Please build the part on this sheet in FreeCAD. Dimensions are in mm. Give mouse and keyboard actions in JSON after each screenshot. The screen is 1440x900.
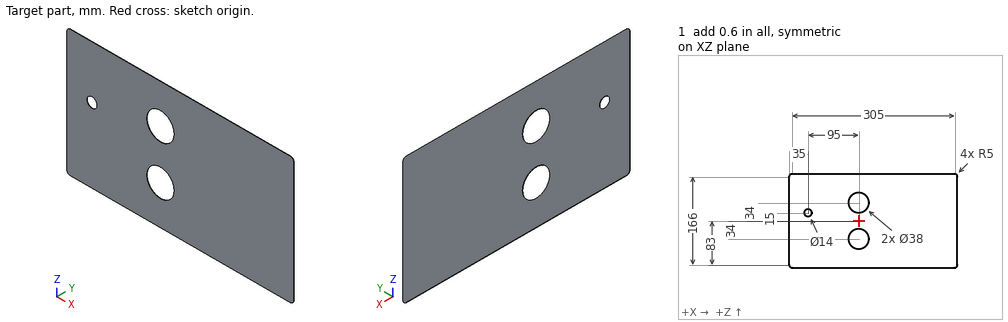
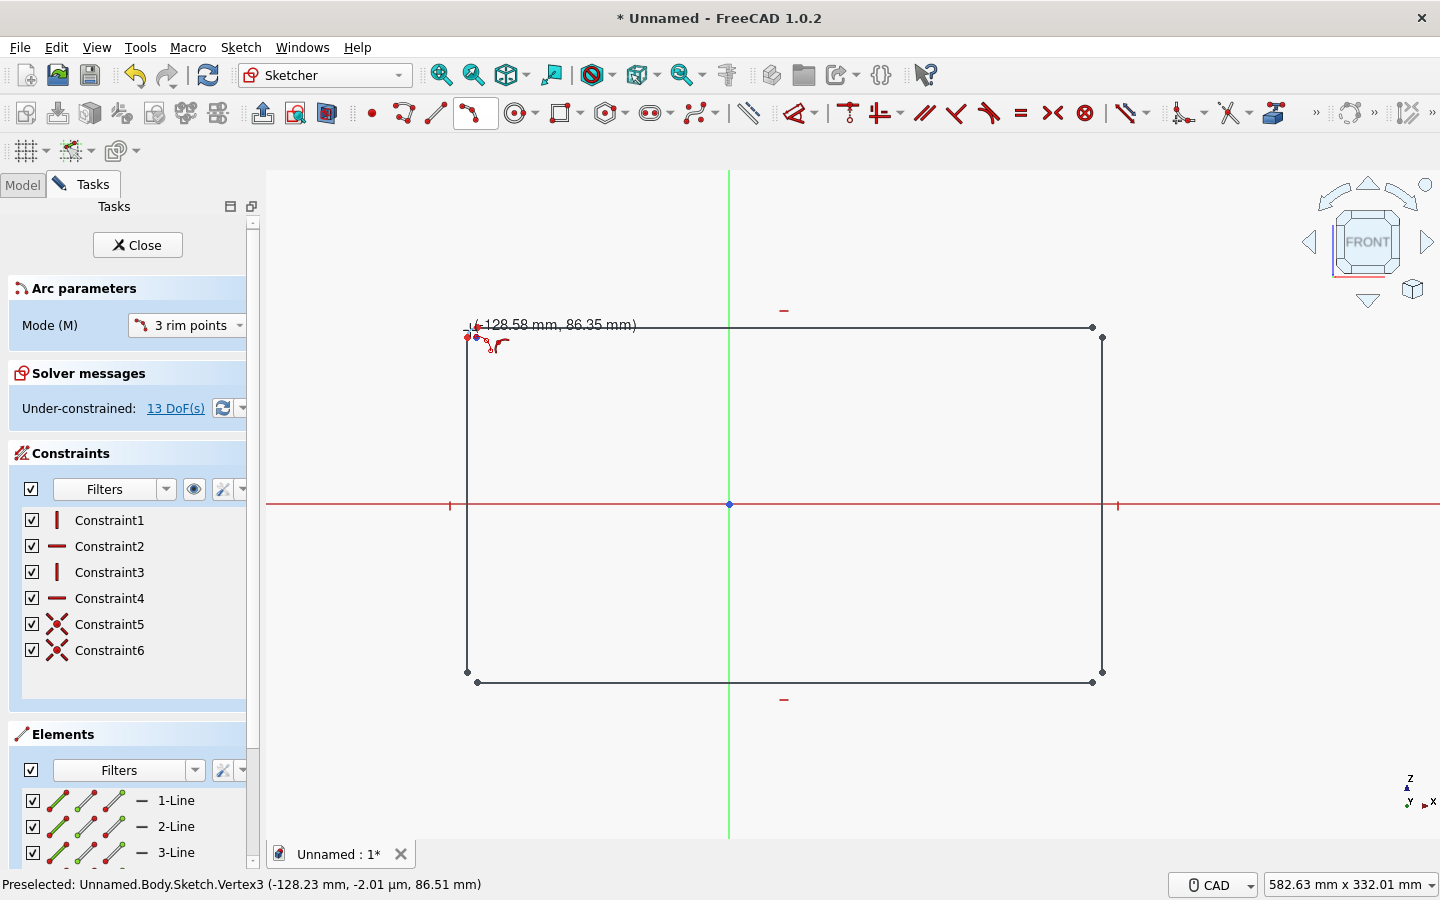
{"action": "left_click", "coordinate": [1092, 328]}
{"action": "left_click", "coordinate": [1102, 338]}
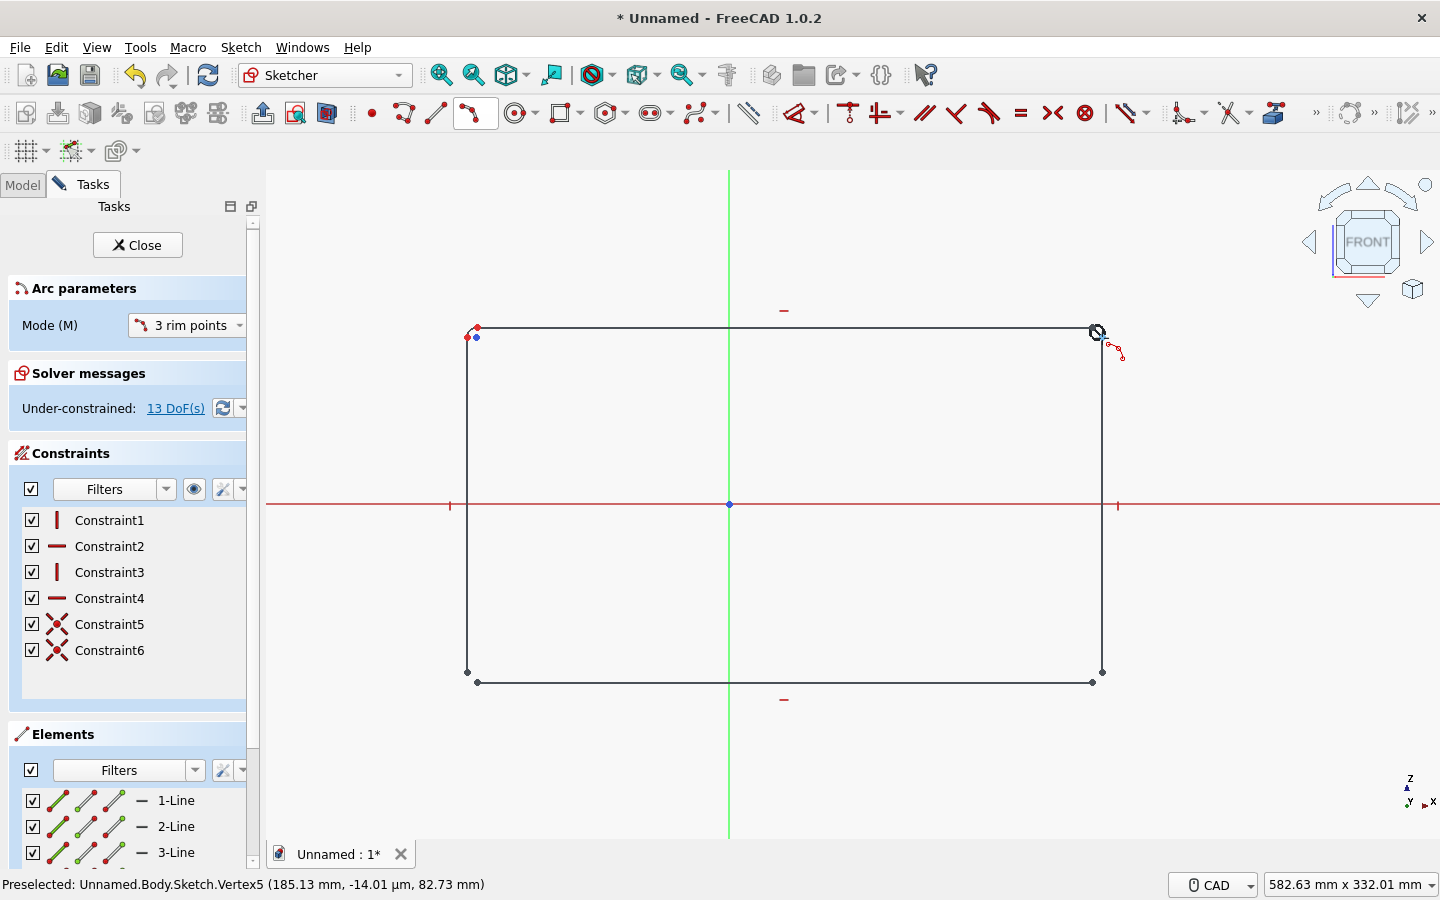
{"action": "scroll", "coordinate": [1099, 330], "scroll_direction": "up", "scroll_amount": 9}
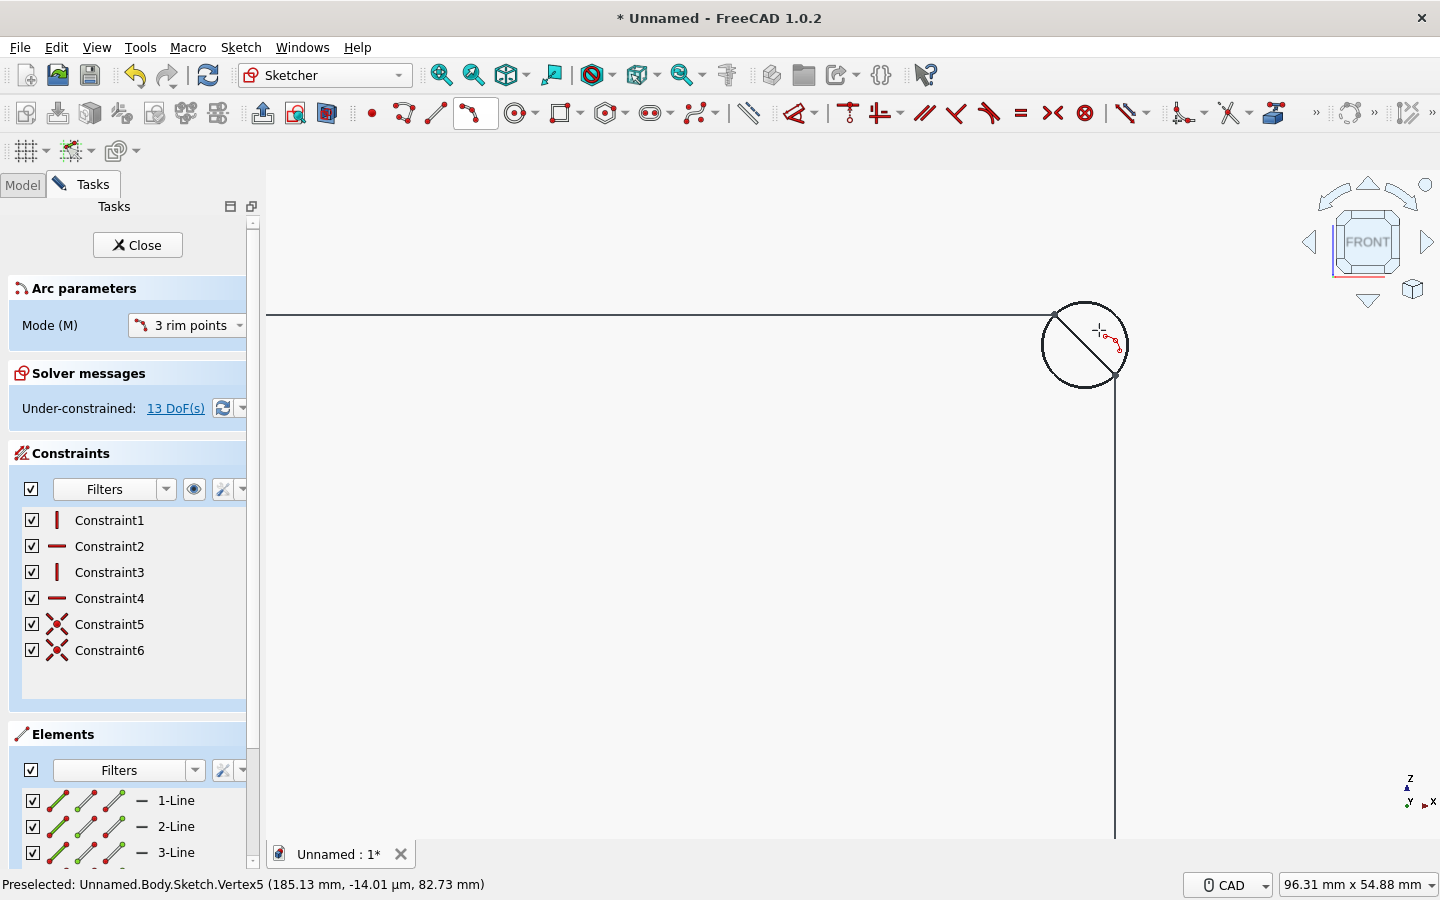
{"action": "left_click", "coordinate": [1096, 329]}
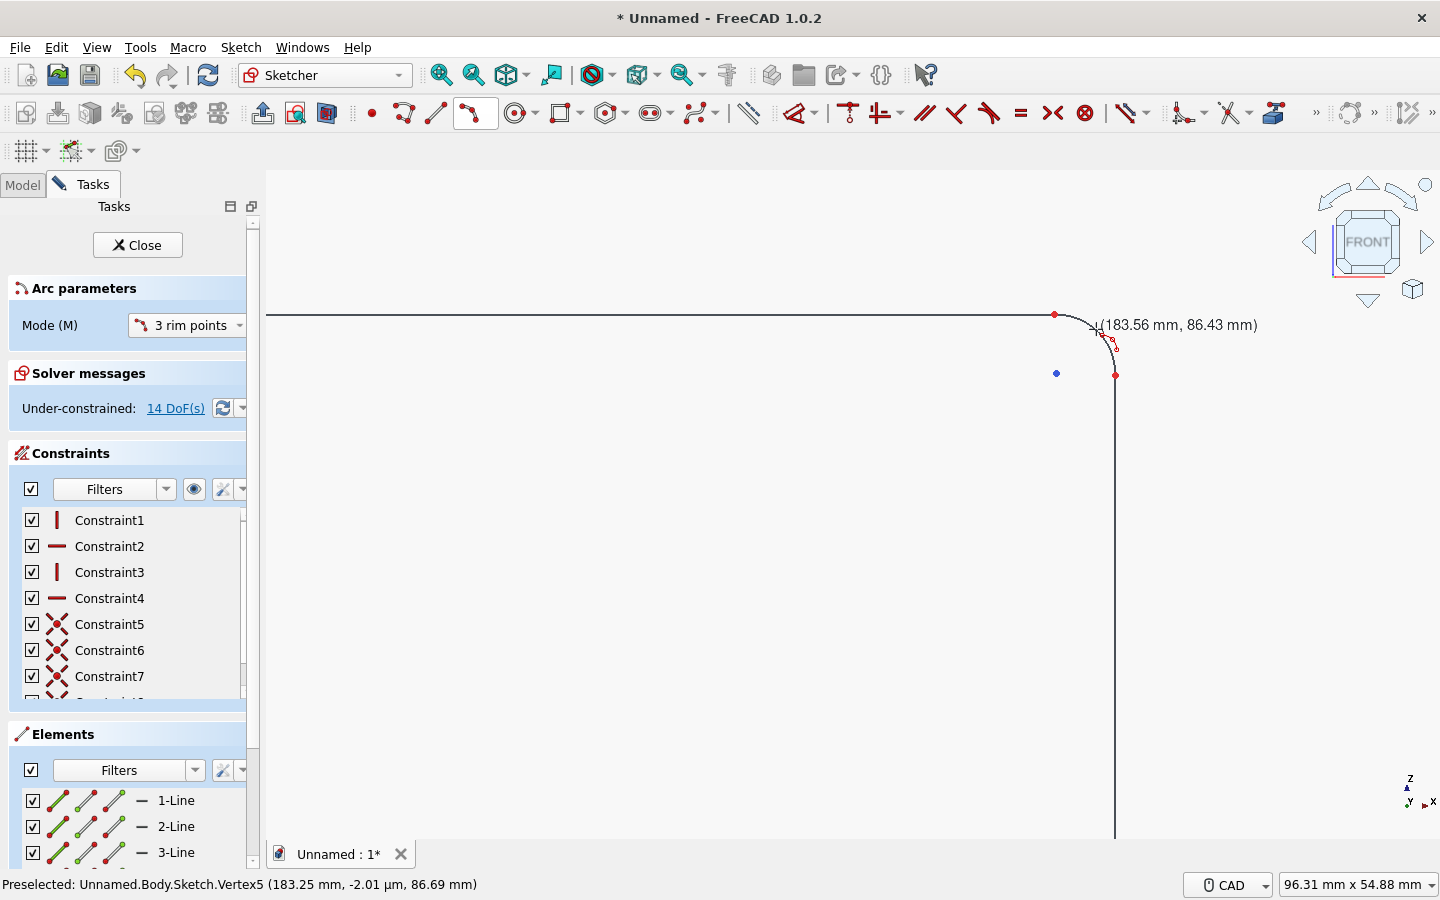
{"action": "scroll", "coordinate": [1100, 330], "scroll_direction": "down", "scroll_amount": 9}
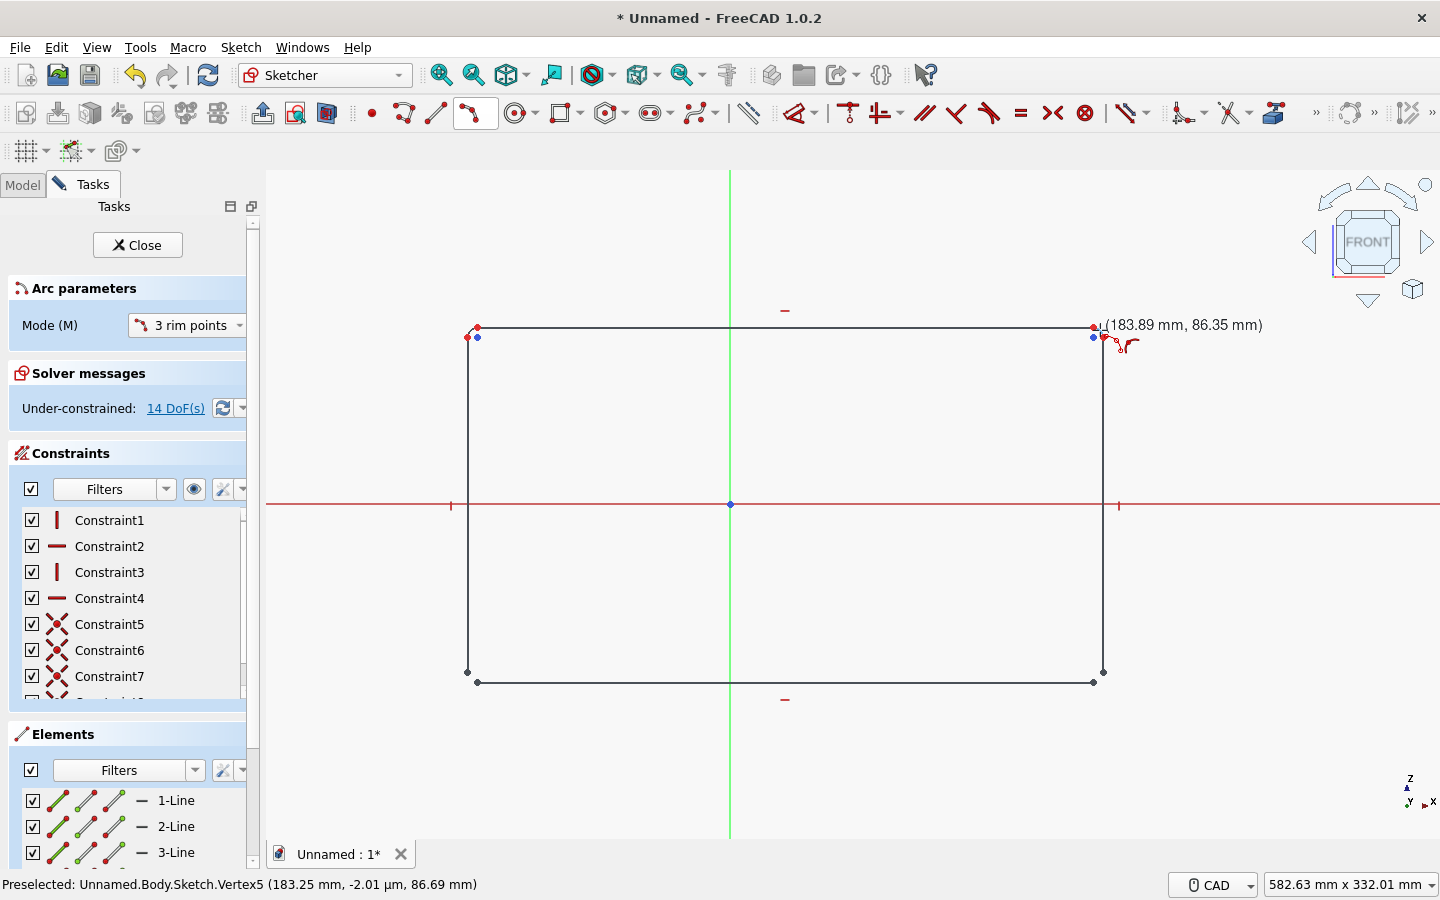
{"action": "left_click", "coordinate": [1103, 673]}
{"action": "left_click", "coordinate": [1093, 683]}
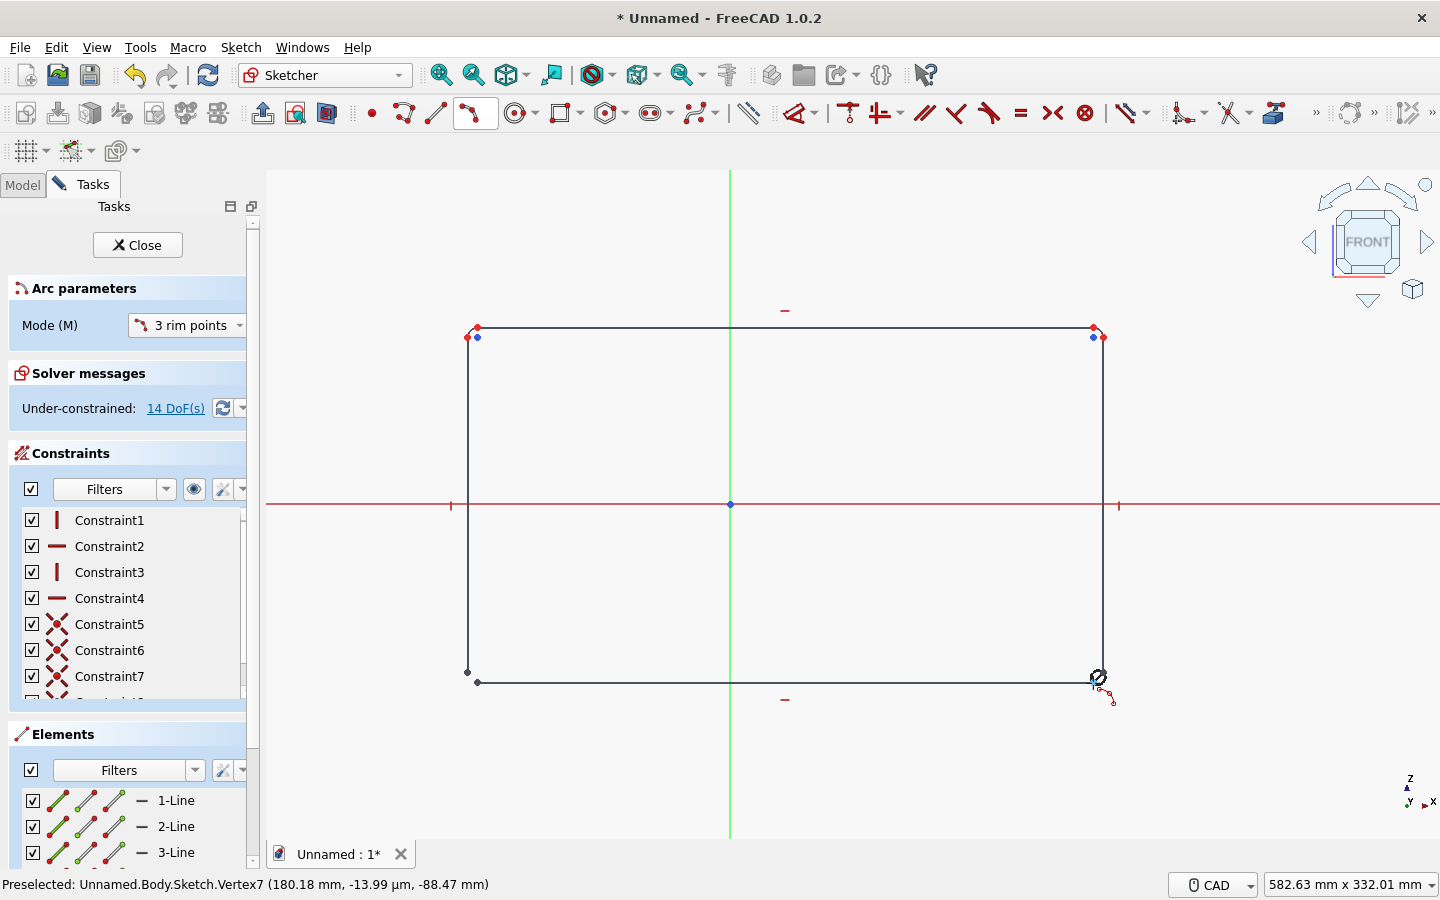
{"action": "scroll", "coordinate": [1100, 679], "scroll_direction": "up", "scroll_amount": 9}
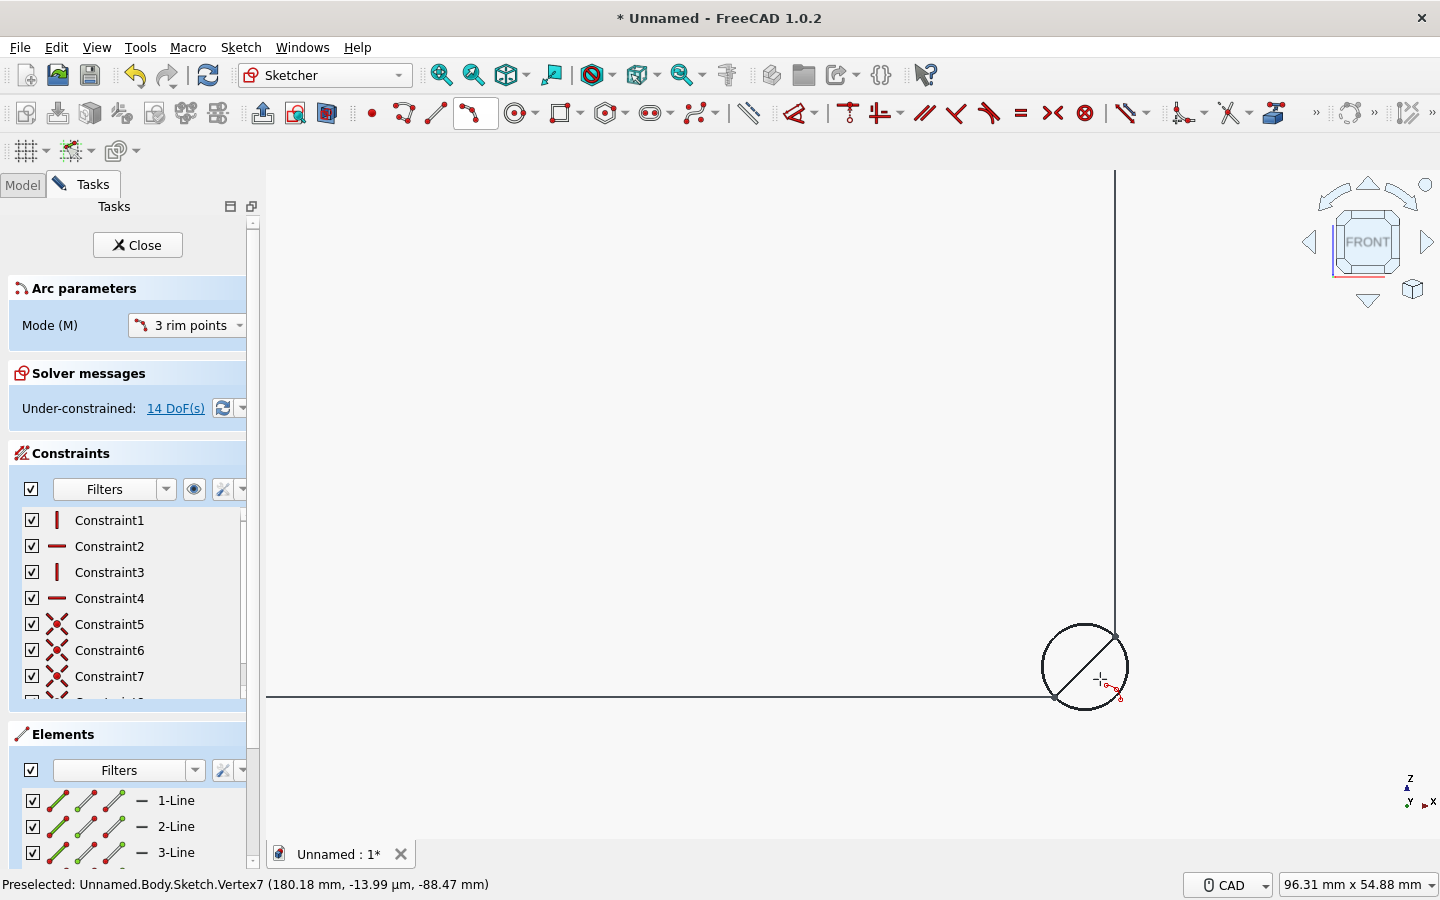
{"action": "left_click", "coordinate": [1096, 674]}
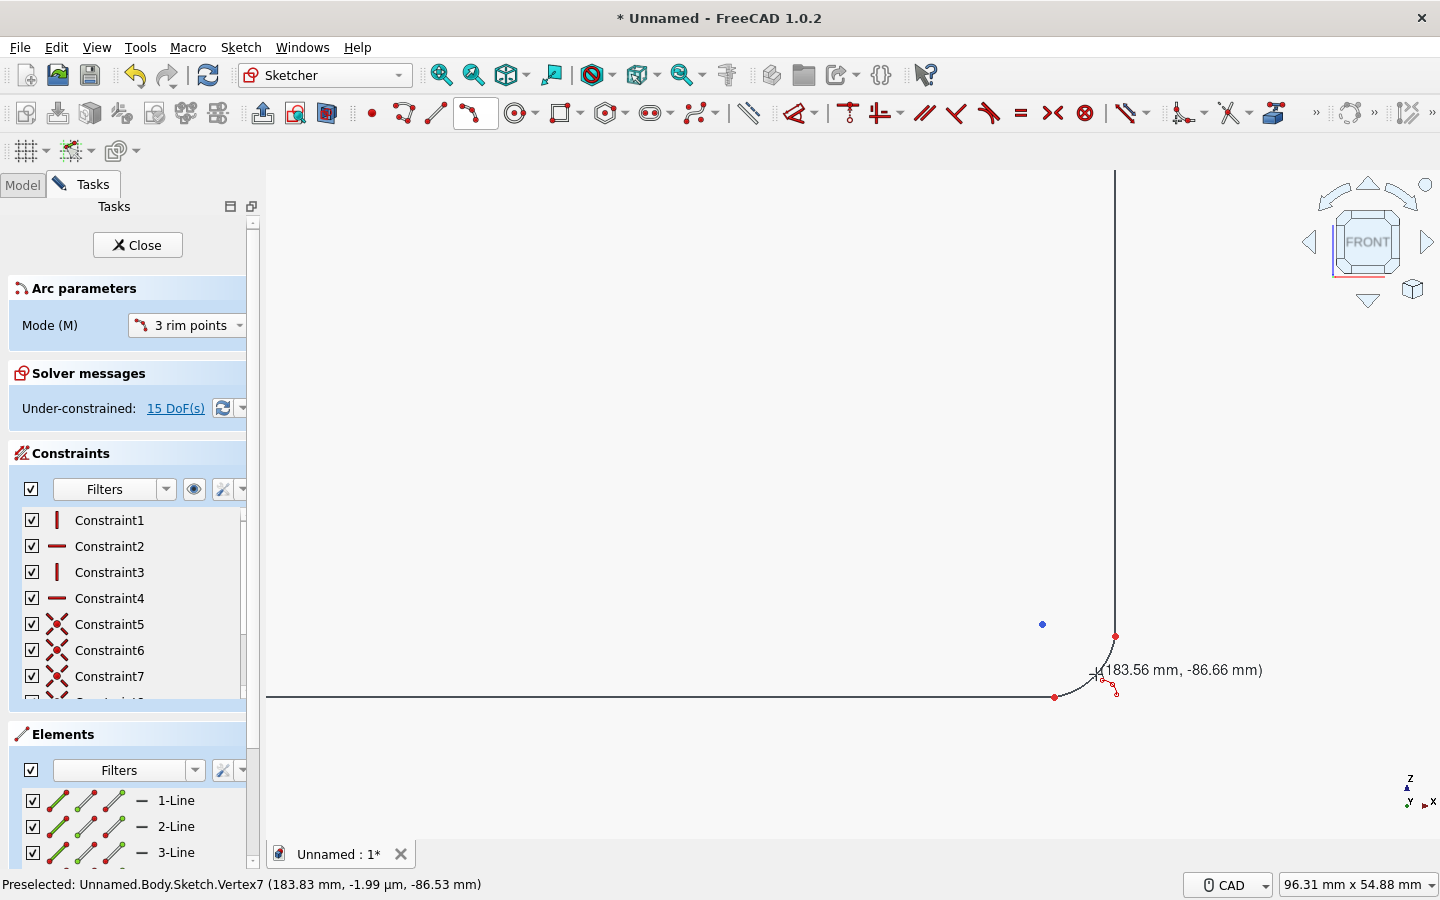
{"action": "scroll", "coordinate": [1100, 680], "scroll_direction": "down", "scroll_amount": 9}